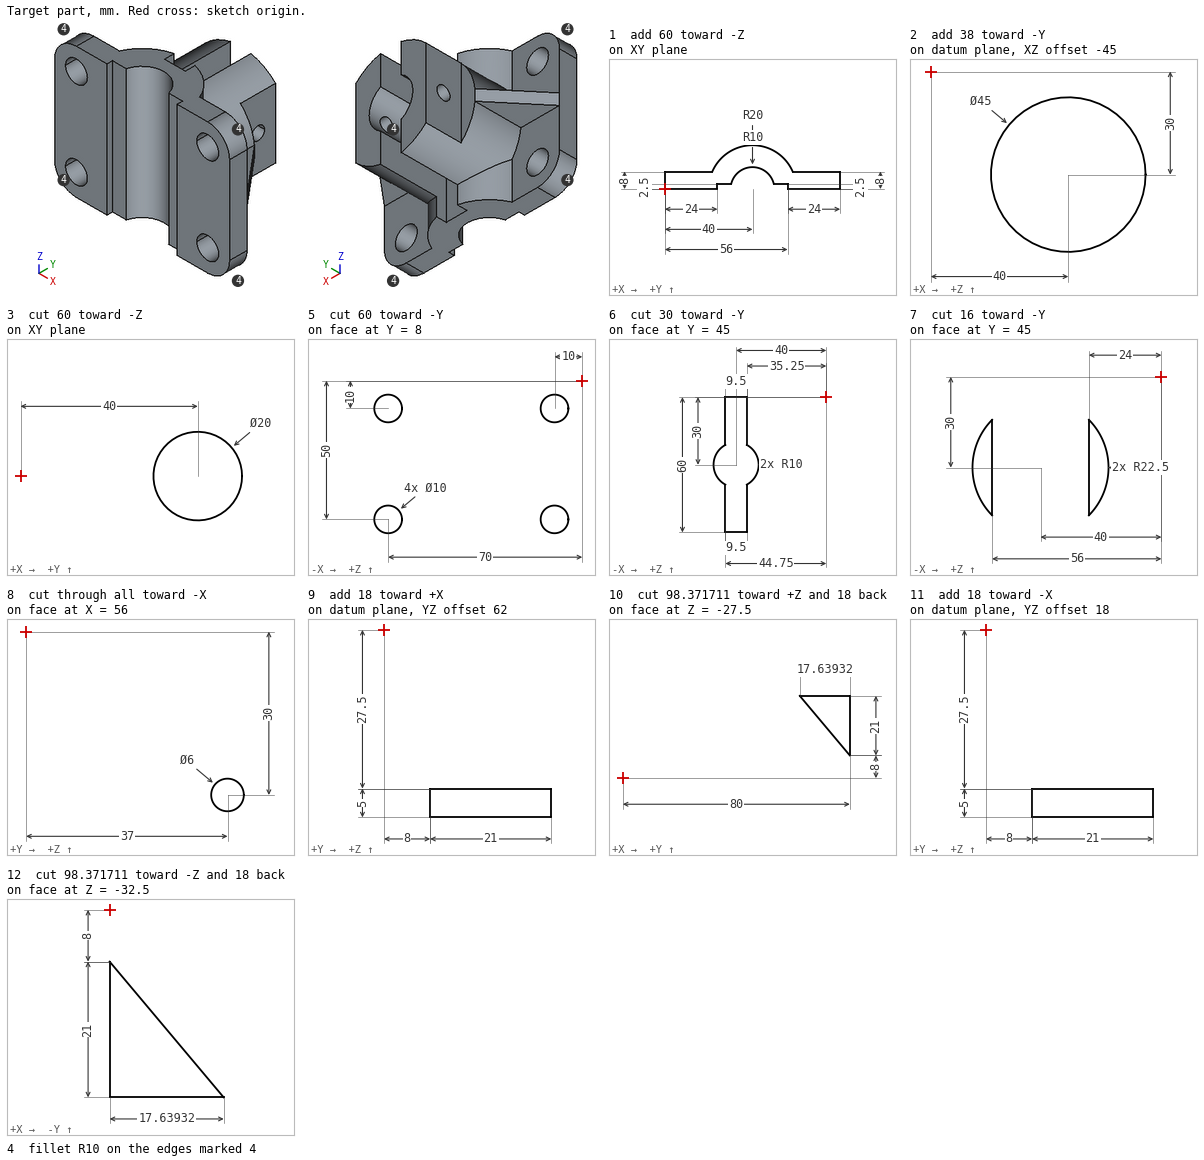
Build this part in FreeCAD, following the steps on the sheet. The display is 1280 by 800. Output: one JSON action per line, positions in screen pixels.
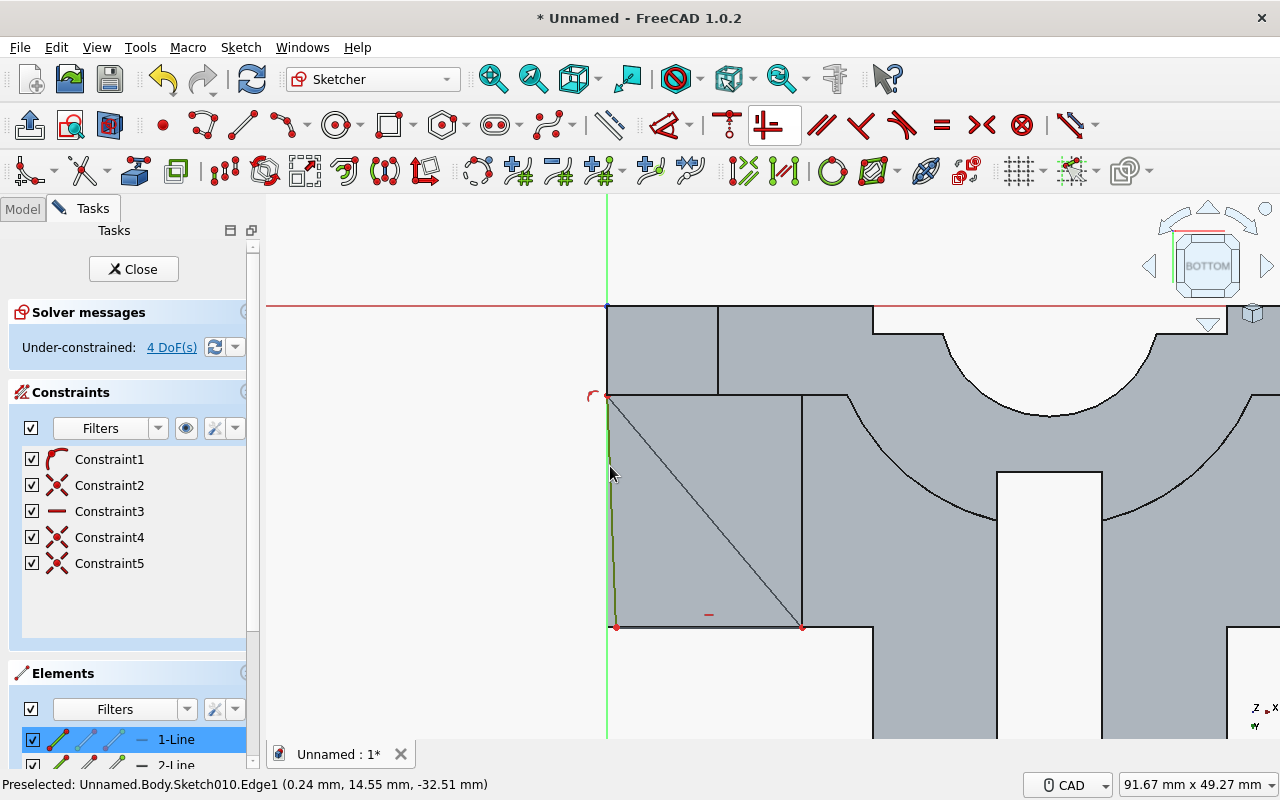
{"action": "left_click", "coordinate": [796, 126]}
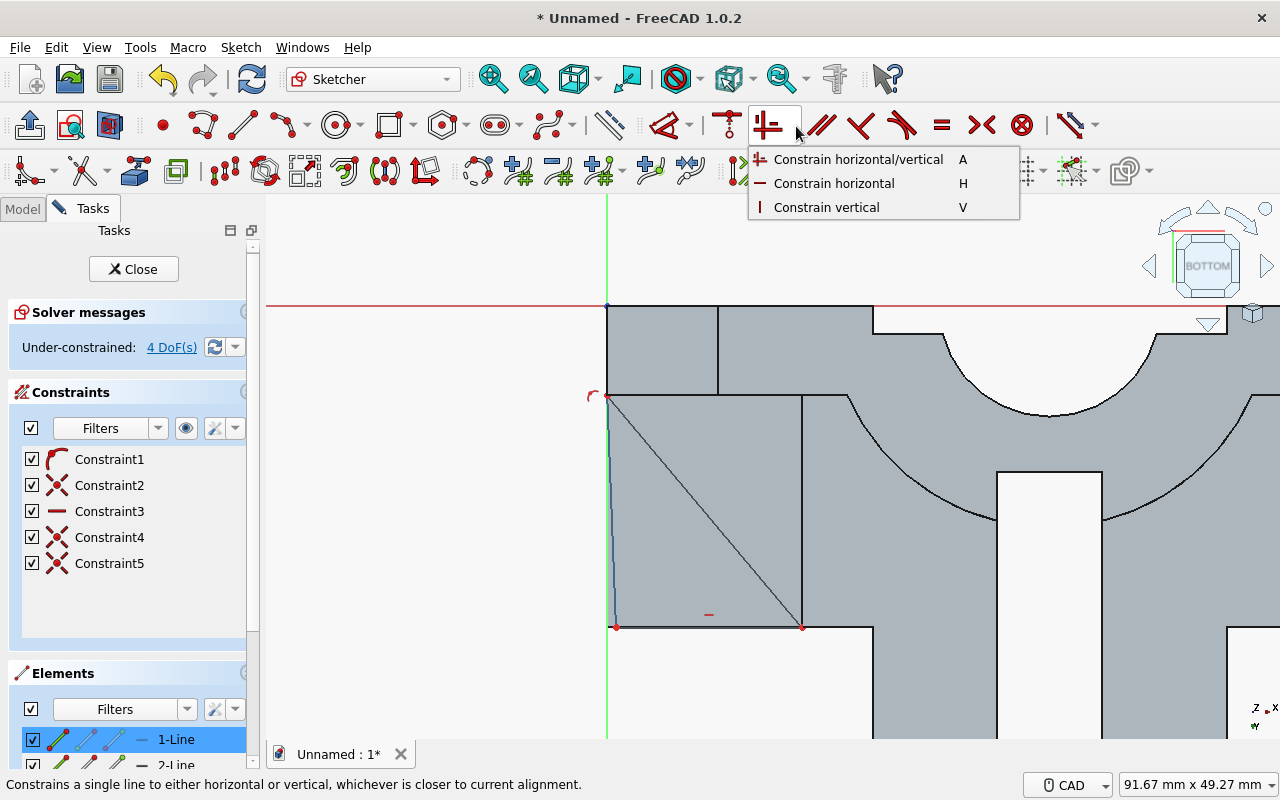
{"action": "left_click", "coordinate": [884, 207]}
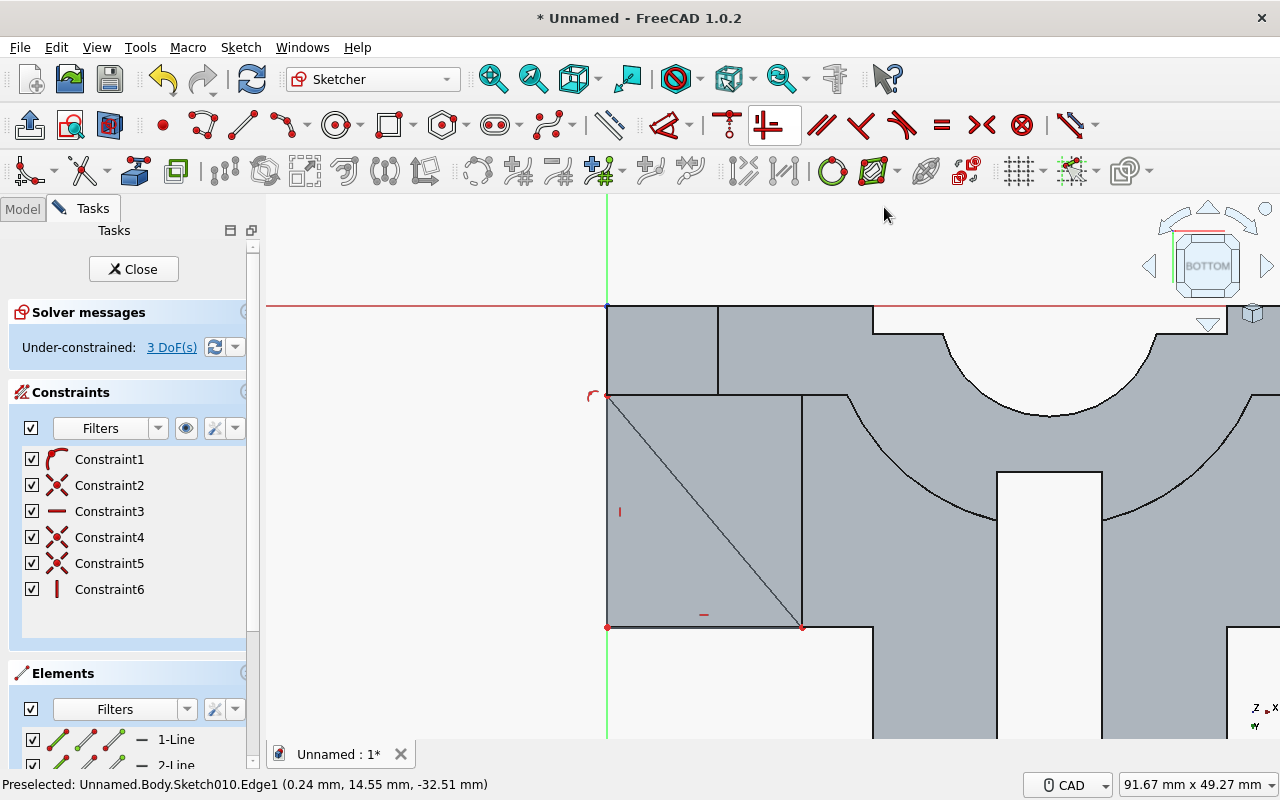
{"action": "left_click", "coordinate": [664, 126]}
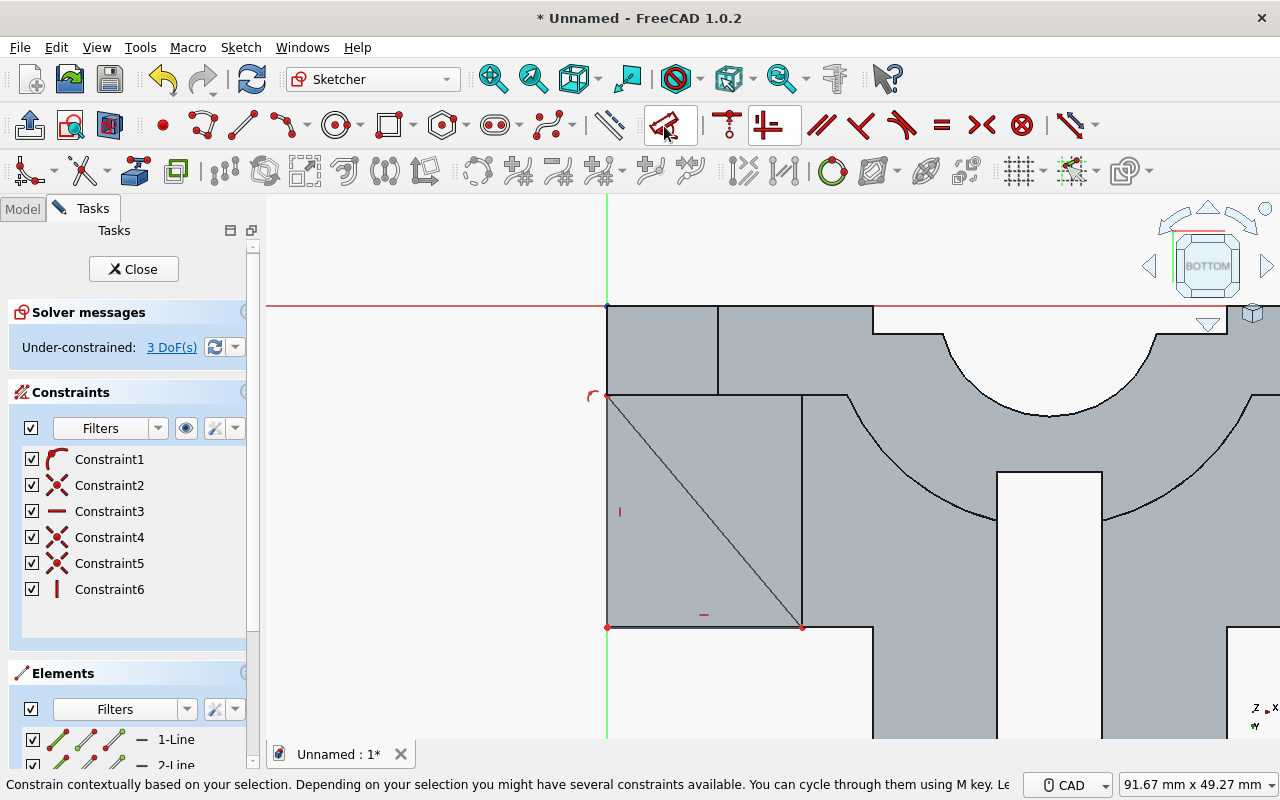
{"action": "left_click", "coordinate": [607, 466]}
{"action": "left_click", "coordinate": [573, 512]}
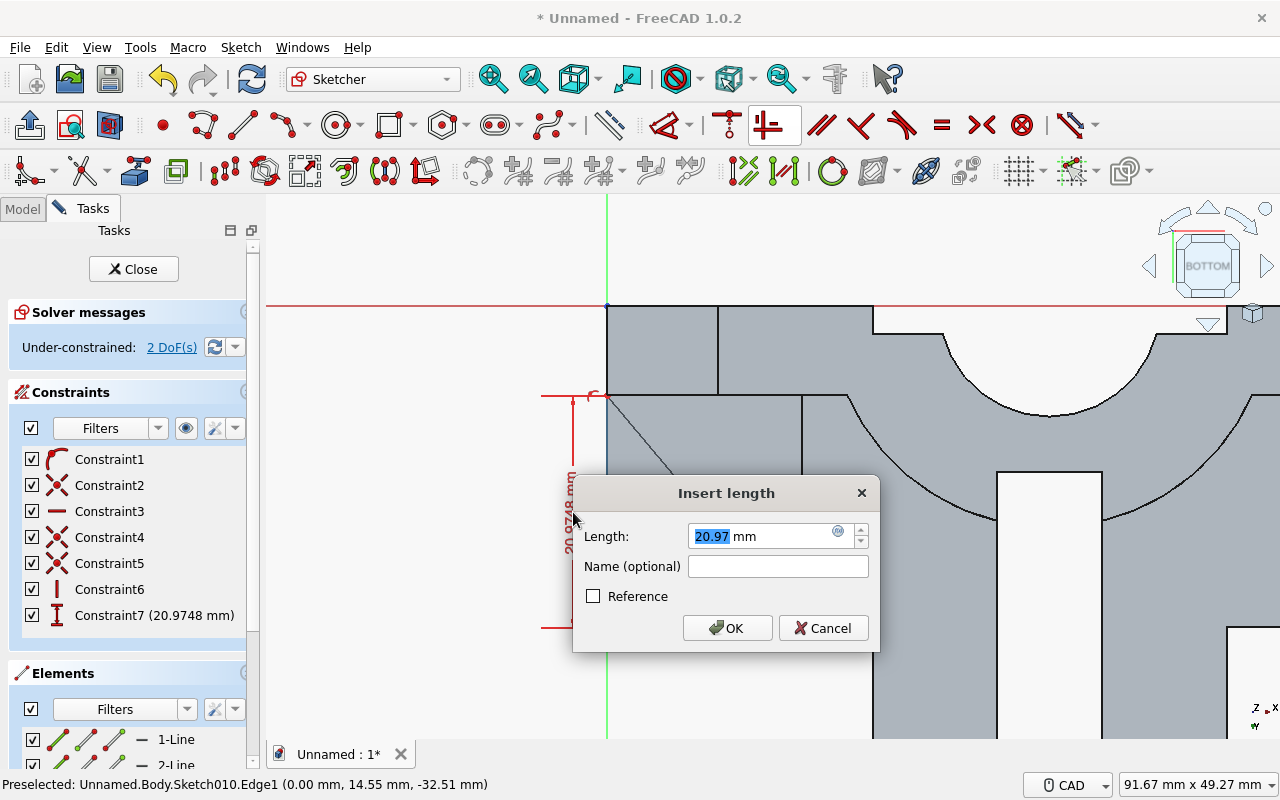
{"action": "type", "text": "21"}
{"action": "key", "text": "Return"}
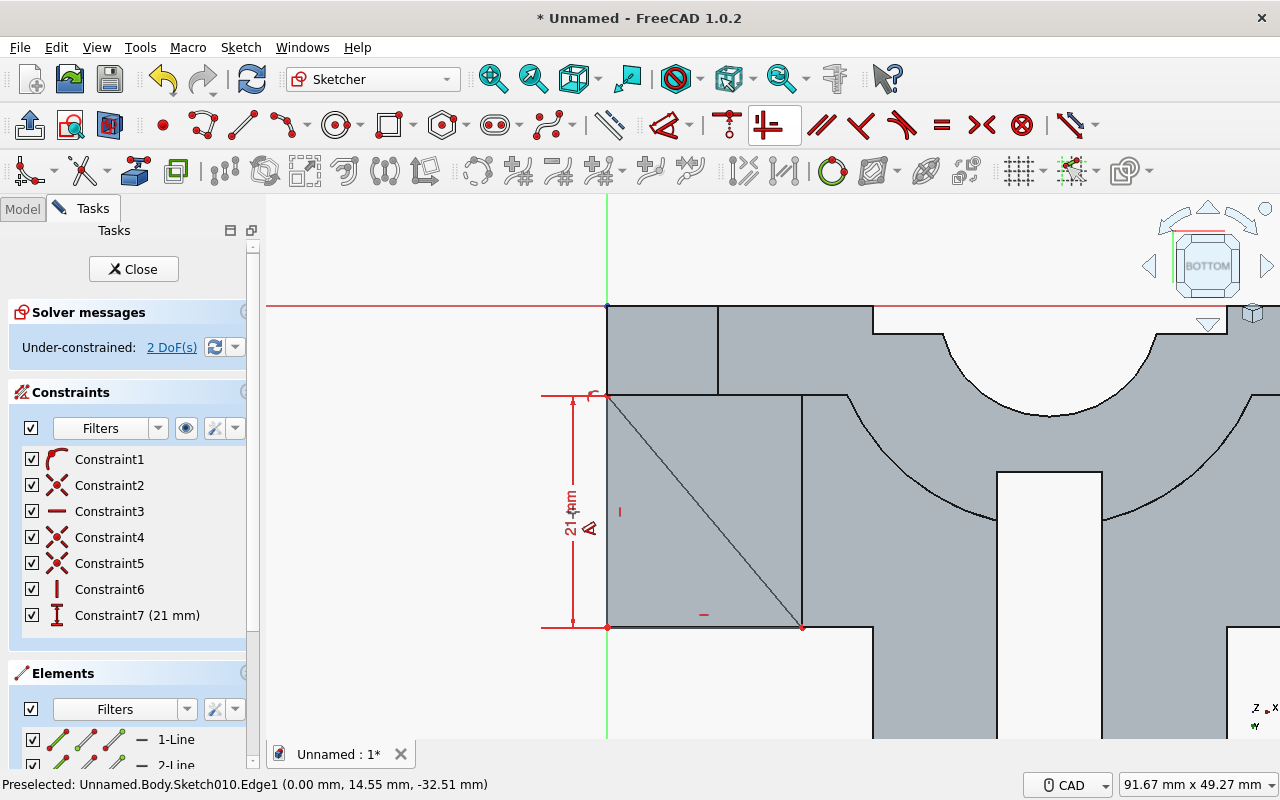
{"action": "left_click", "coordinate": [607, 396]}
{"action": "left_click", "coordinate": [573, 351]}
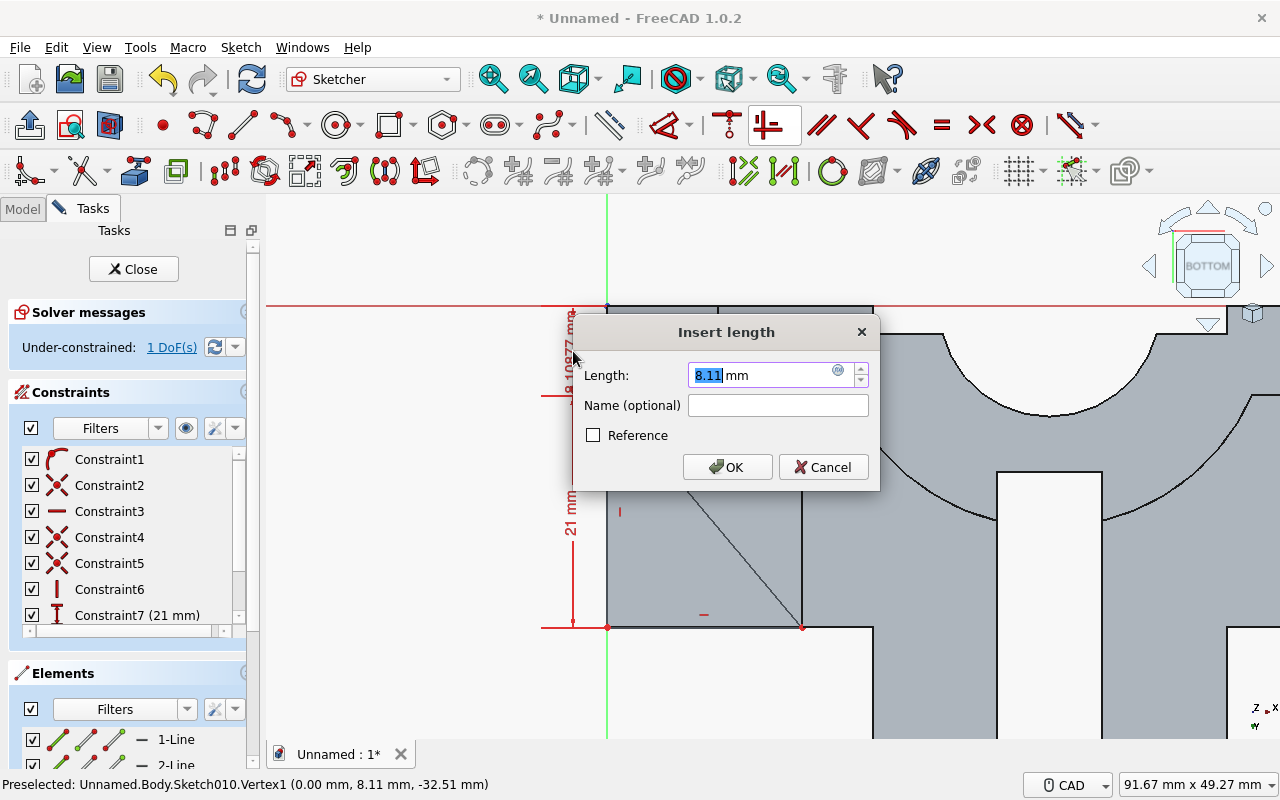
{"action": "type", "text": "8"}
{"action": "key", "text": "Return"}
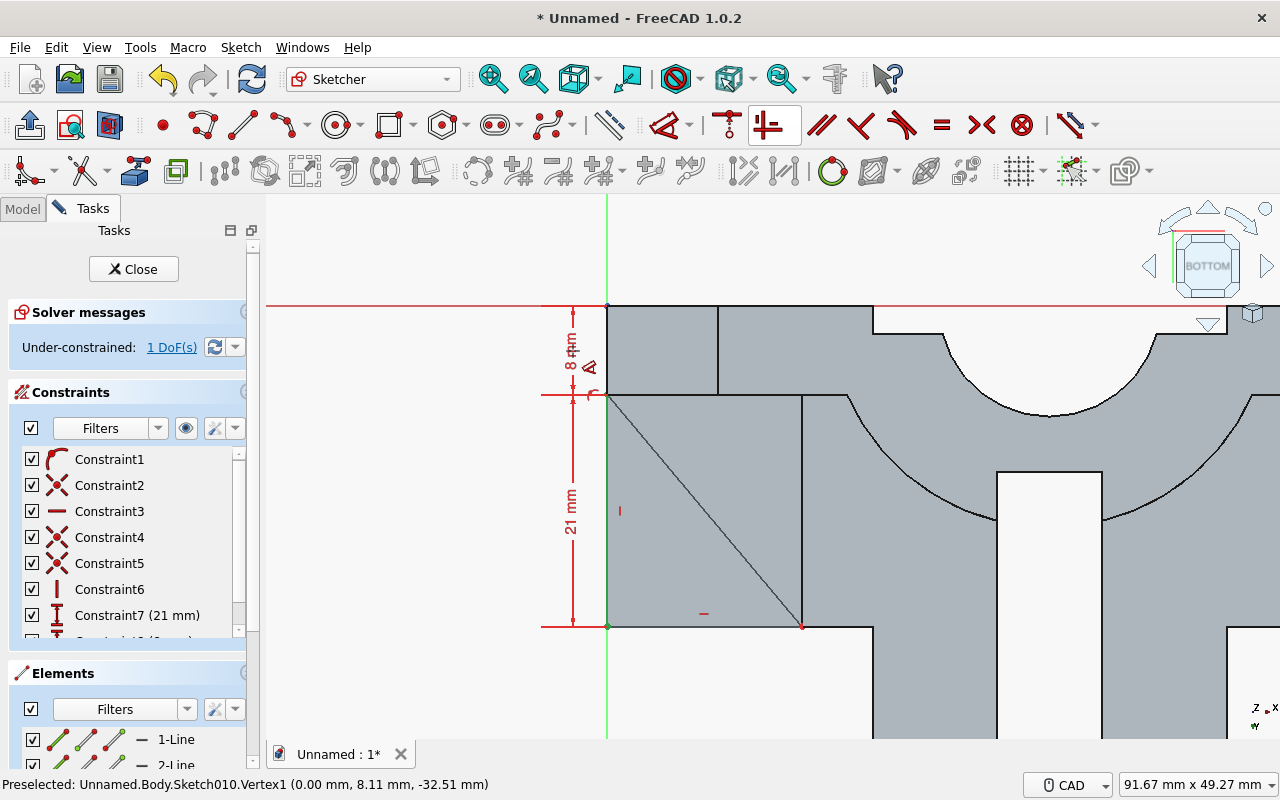
{"action": "left_click", "coordinate": [666, 627]}
{"action": "left_click", "coordinate": [705, 661]}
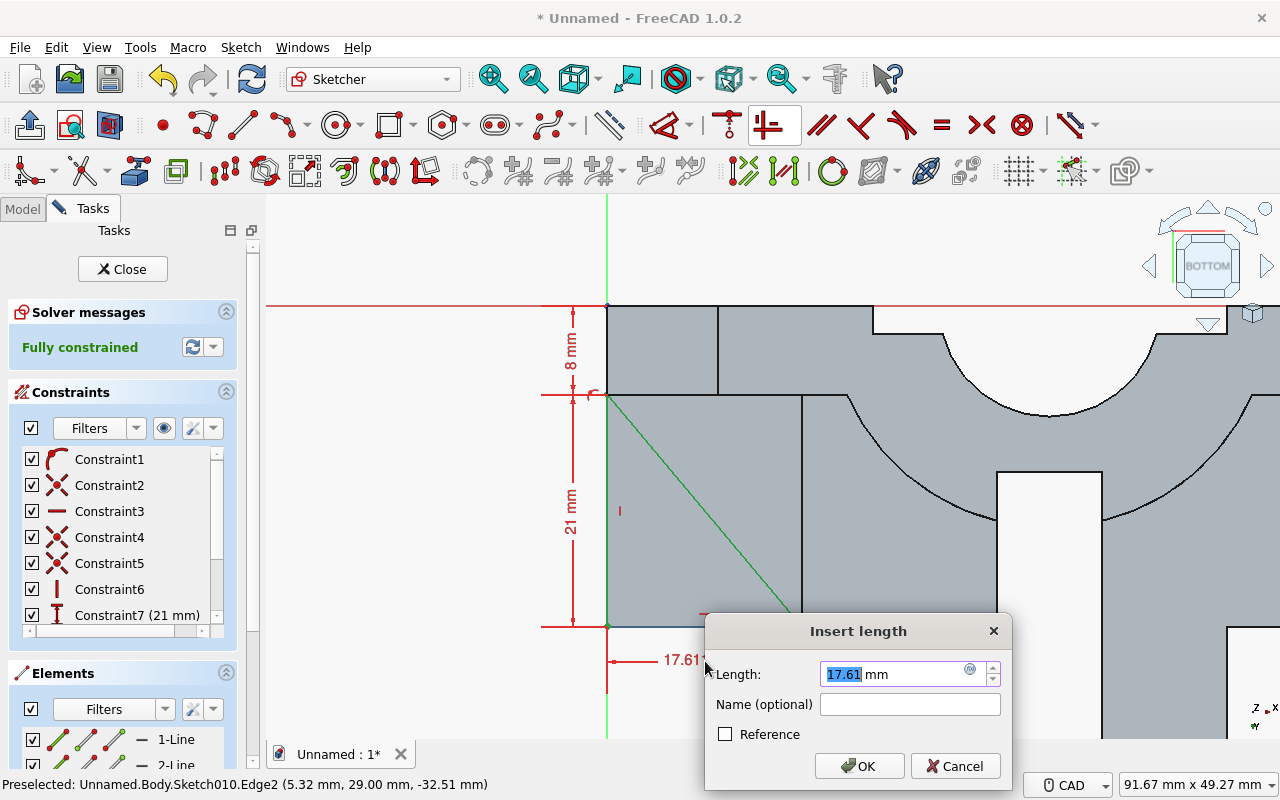
{"action": "type", "text": "17.63932"}
{"action": "key", "text": "Return"}
{"action": "key", "text": "Escape"}